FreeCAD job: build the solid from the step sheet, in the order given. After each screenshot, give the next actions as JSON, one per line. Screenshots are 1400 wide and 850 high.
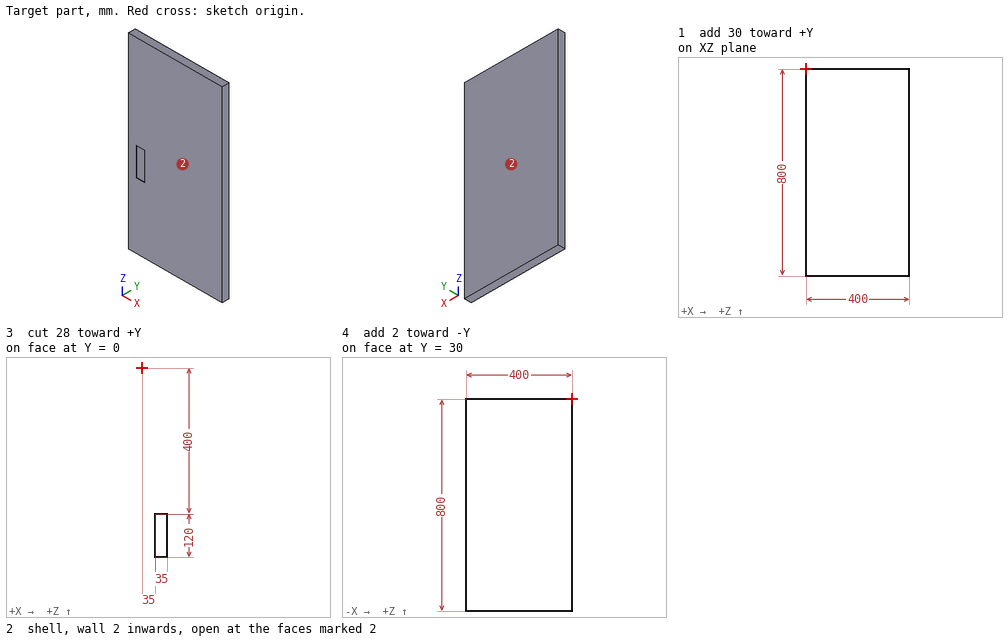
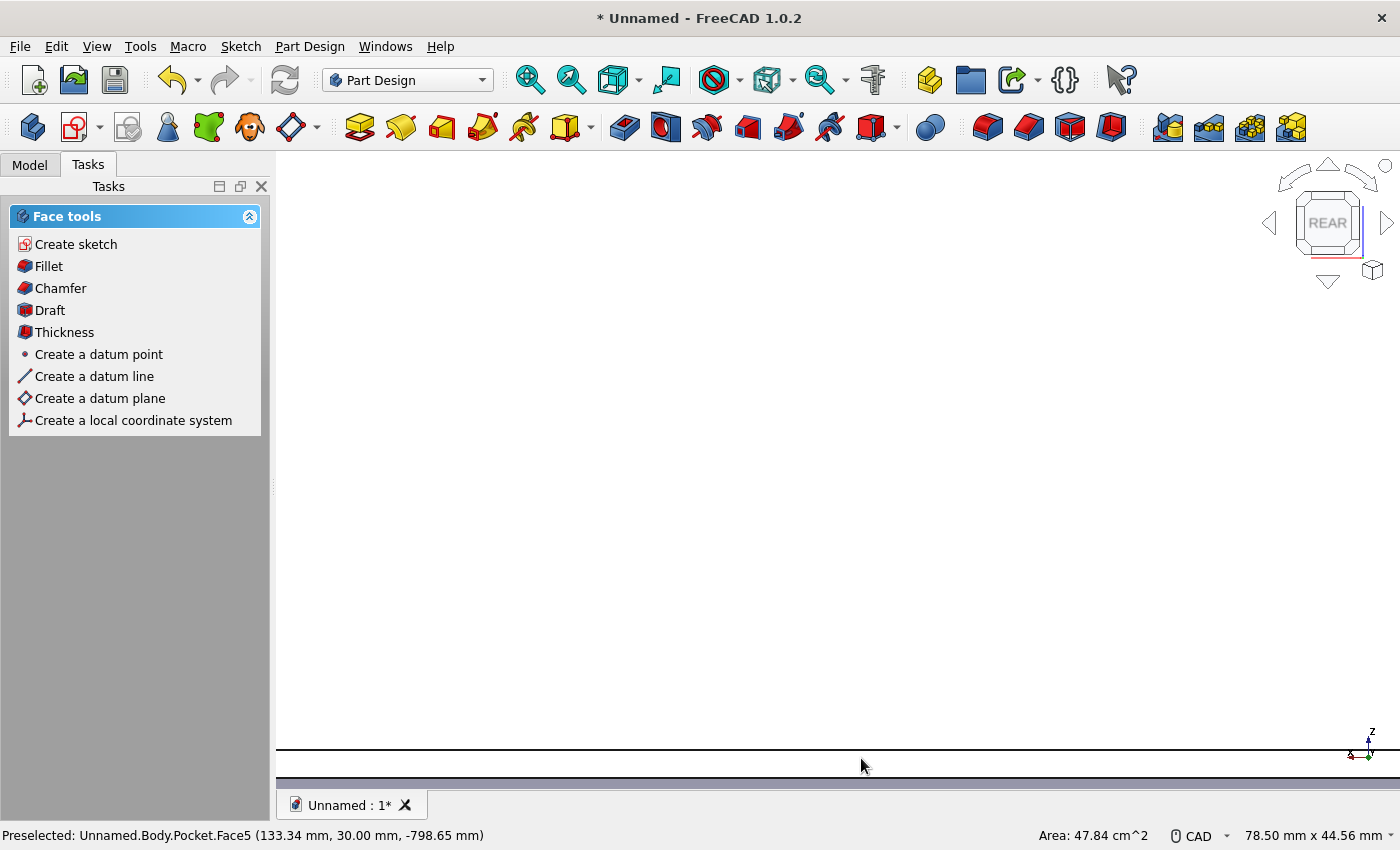
{"action": "left_click", "coordinate": [74, 128]}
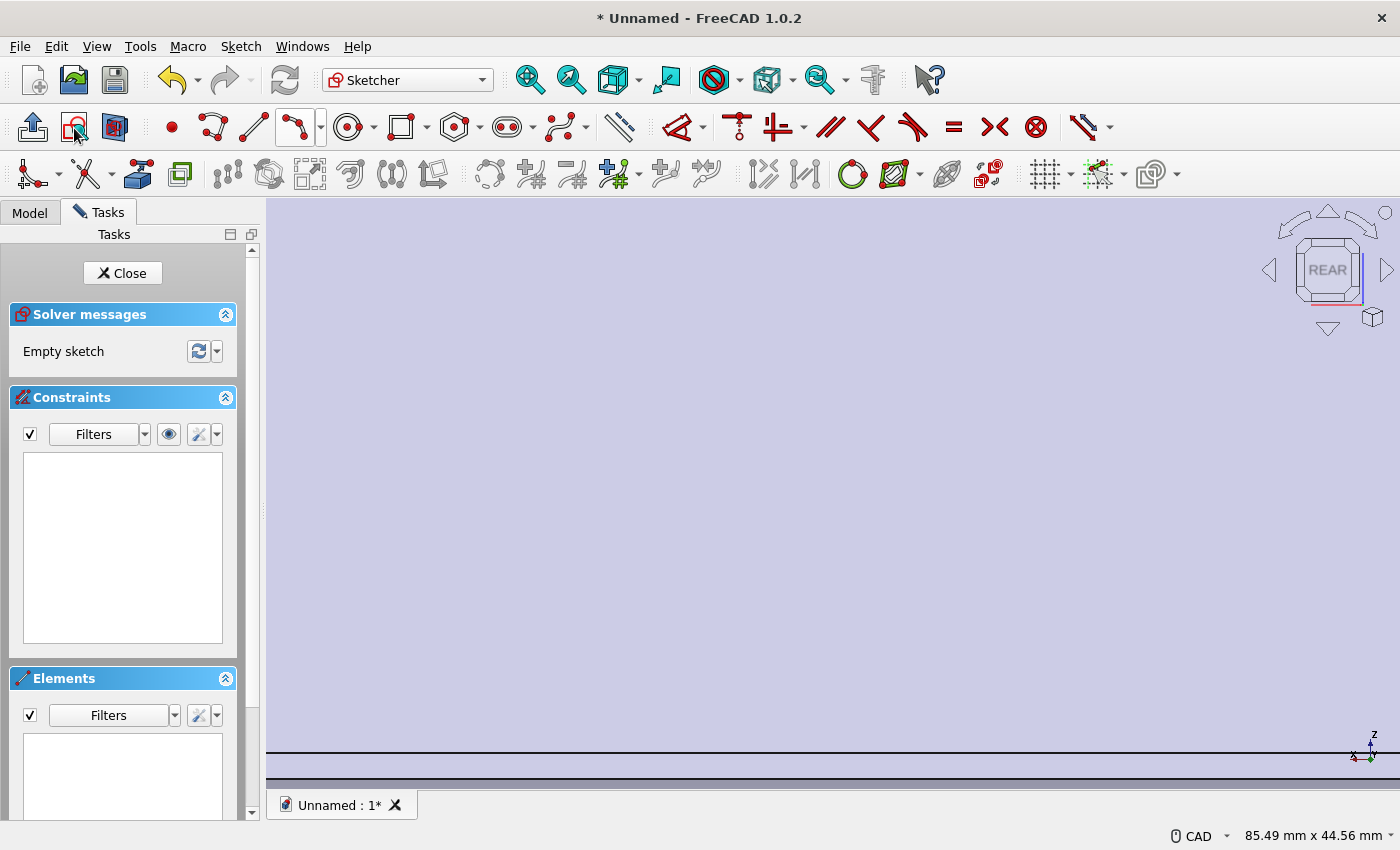
{"action": "scroll", "coordinate": [798, 707], "scroll_direction": "down", "scroll_amount": 16}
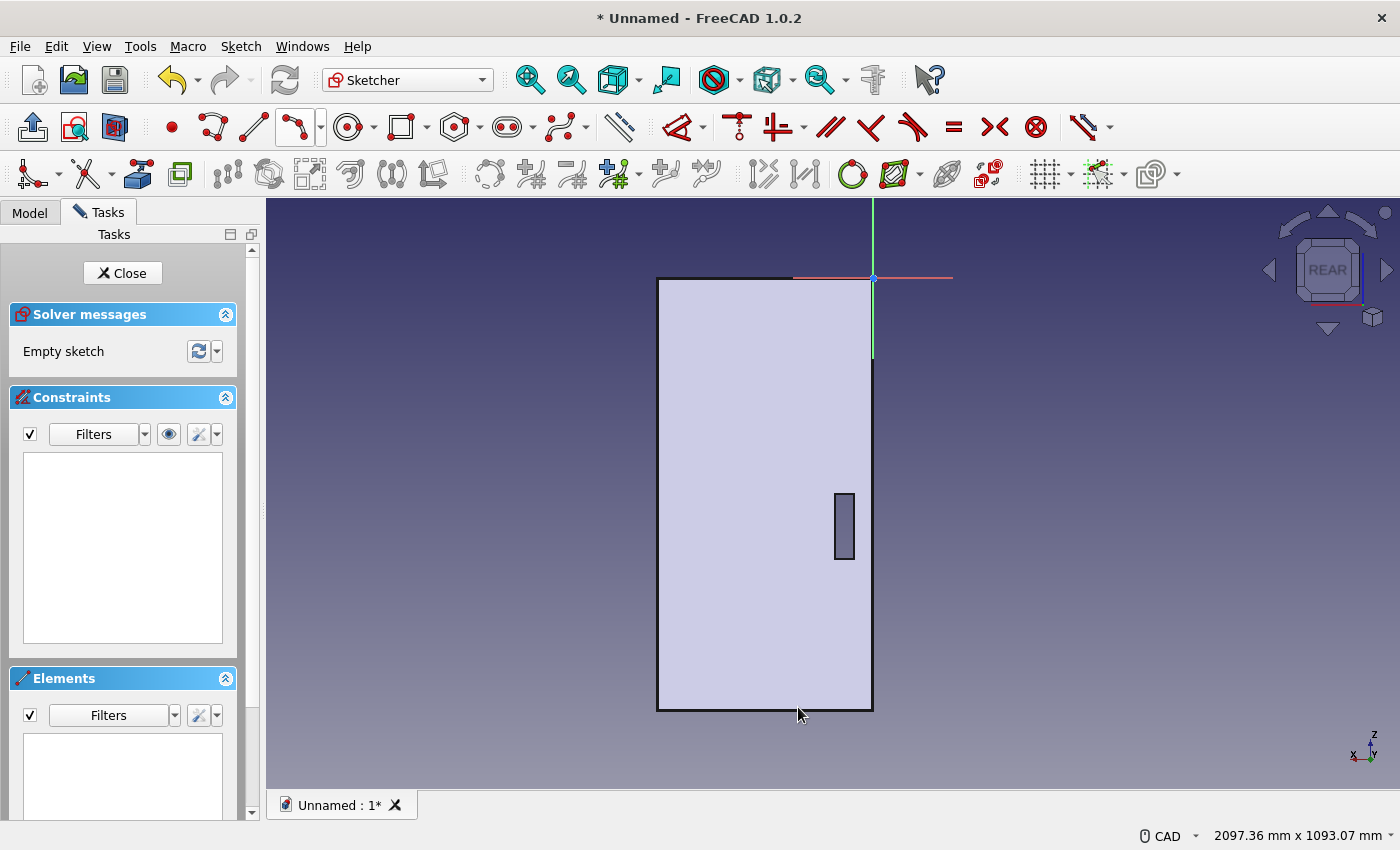
{"action": "key", "text": "g r"}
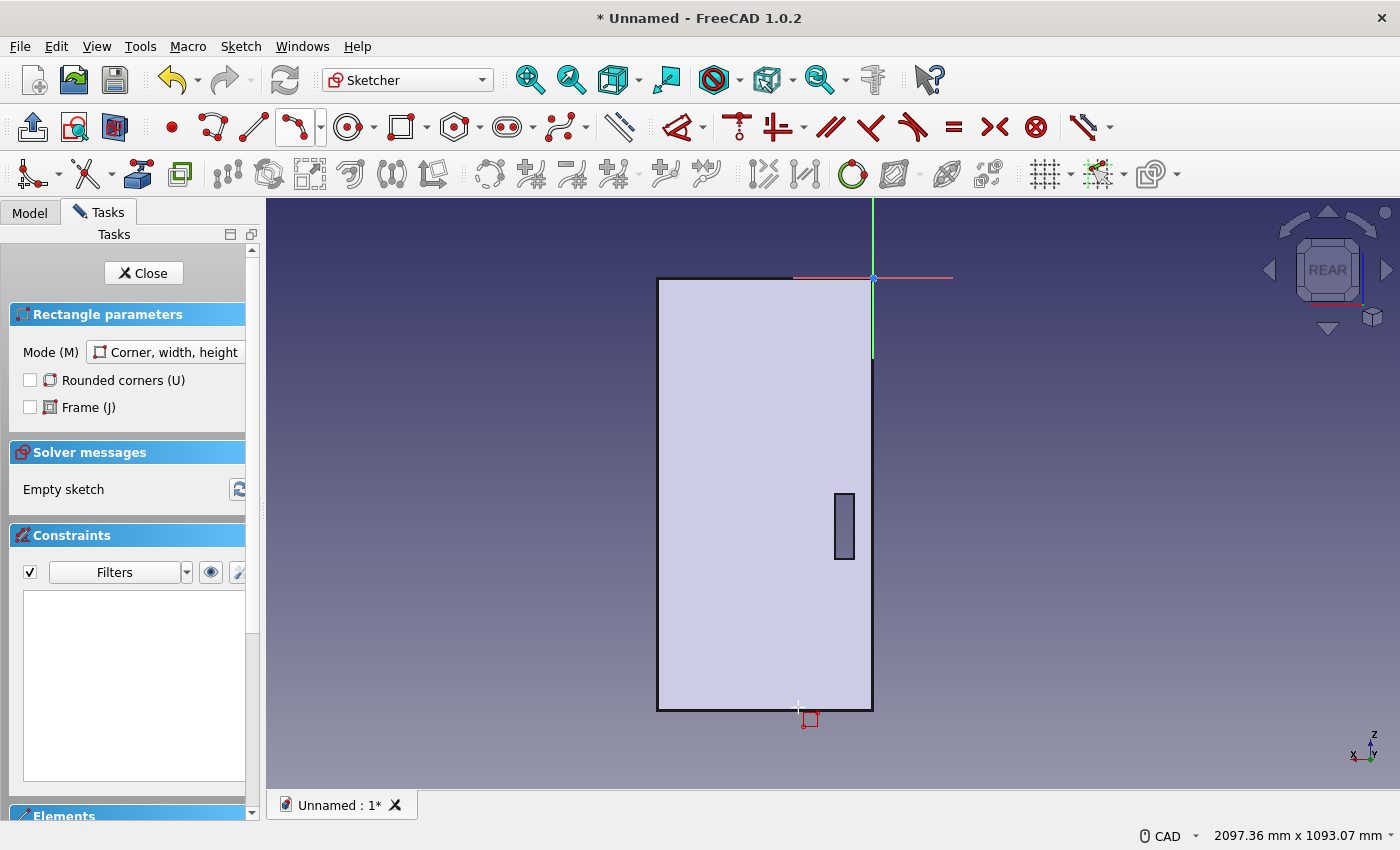
{"action": "left_click", "coordinate": [873, 278]}
{"action": "left_click", "coordinate": [657, 711]}
{"action": "key", "text": "Escape"}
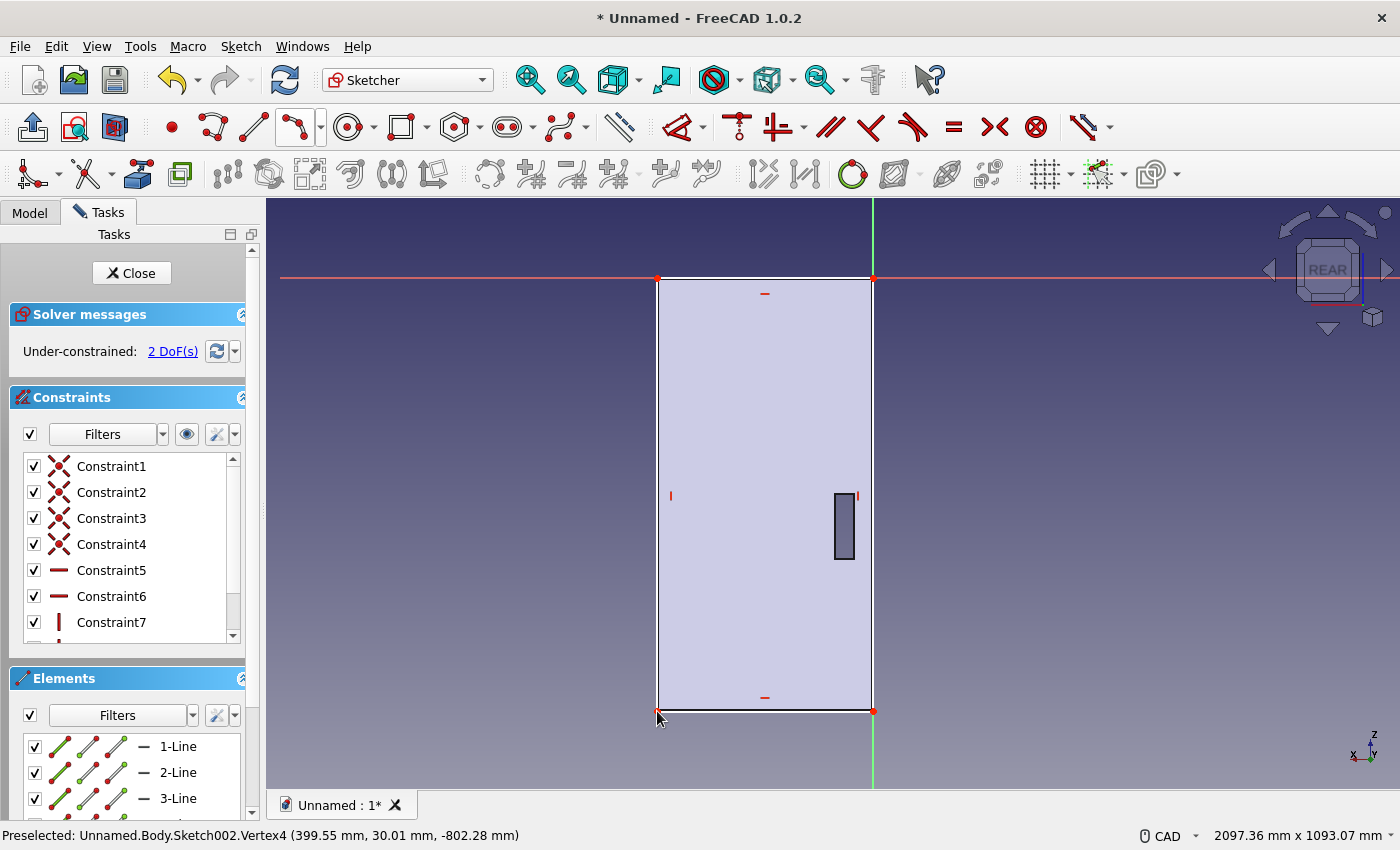
{"action": "left_click", "coordinate": [676, 128]}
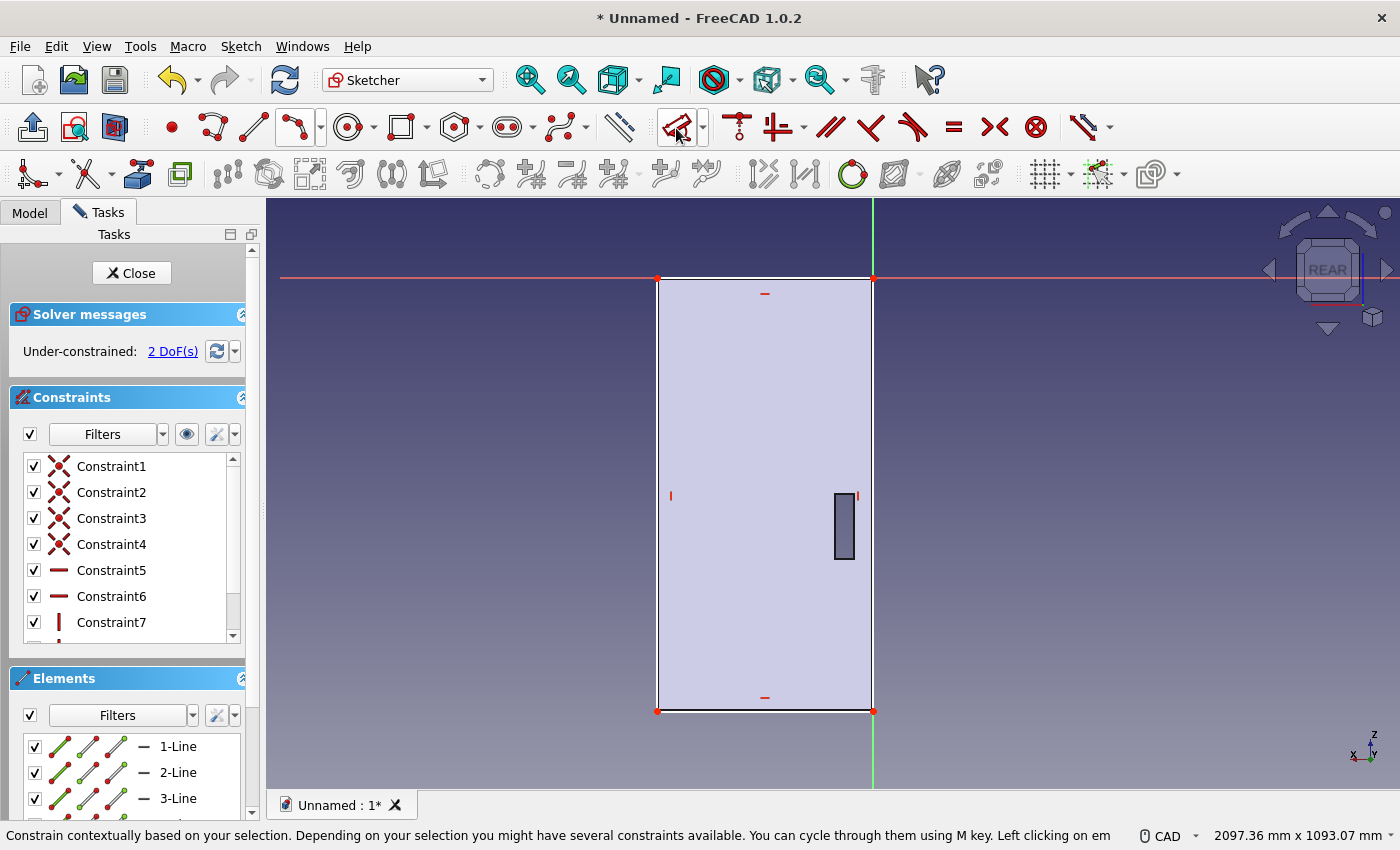
{"action": "left_click", "coordinate": [808, 278]}
{"action": "left_click", "coordinate": [765, 244]}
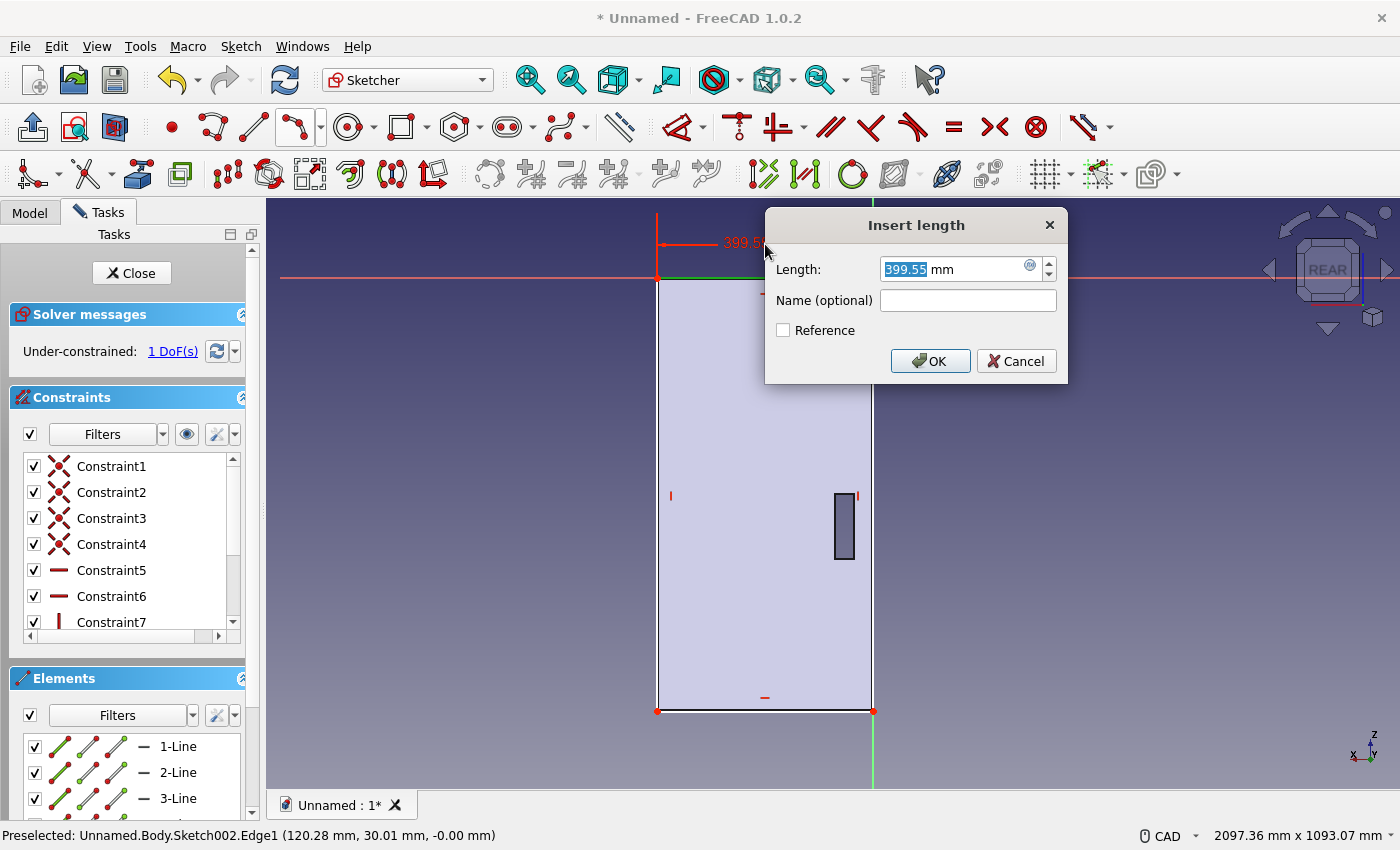
{"action": "type", "text": "400"}
{"action": "key", "text": "Return"}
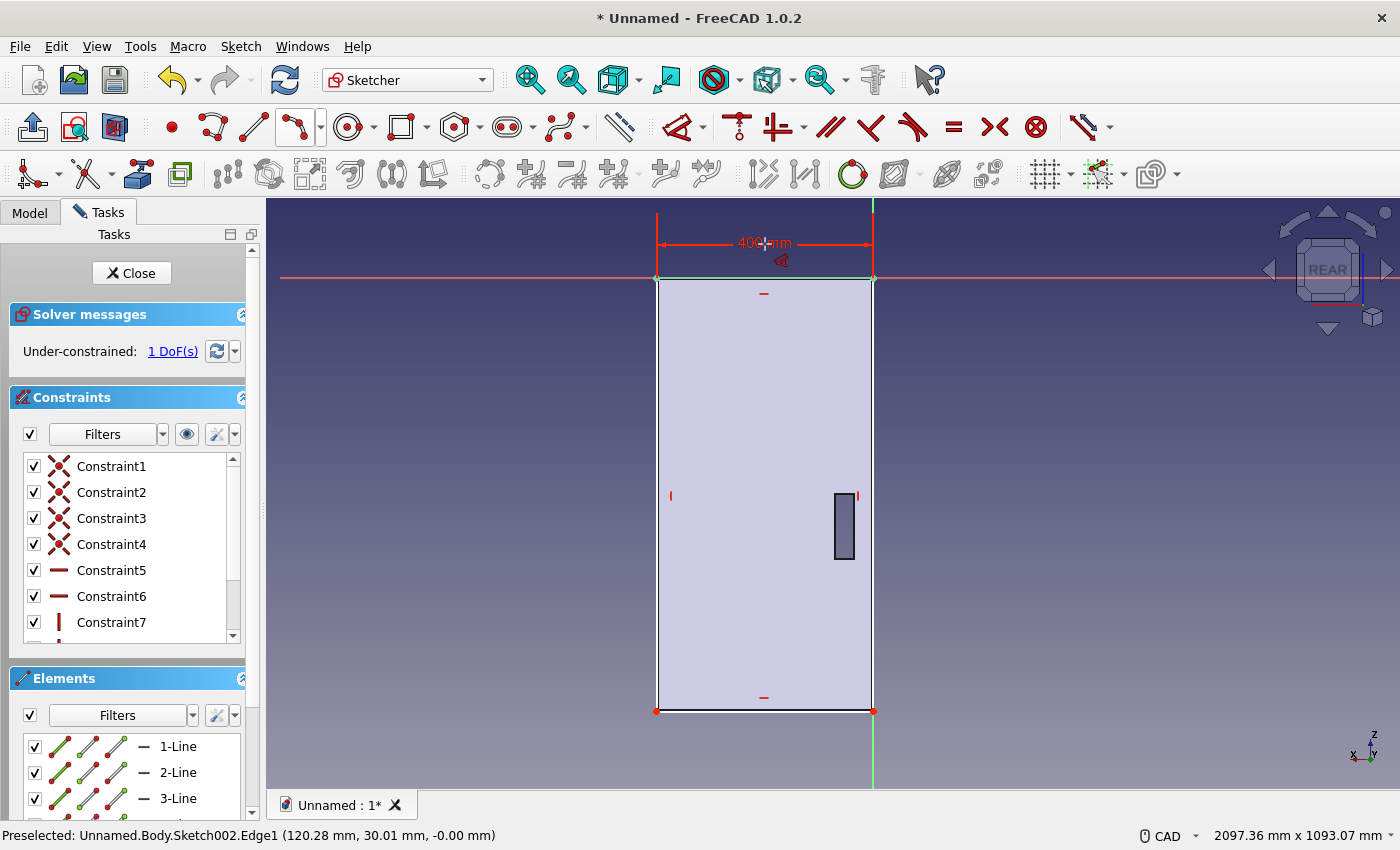
{"action": "left_click", "coordinate": [657, 408]}
{"action": "left_click", "coordinate": [623, 495]}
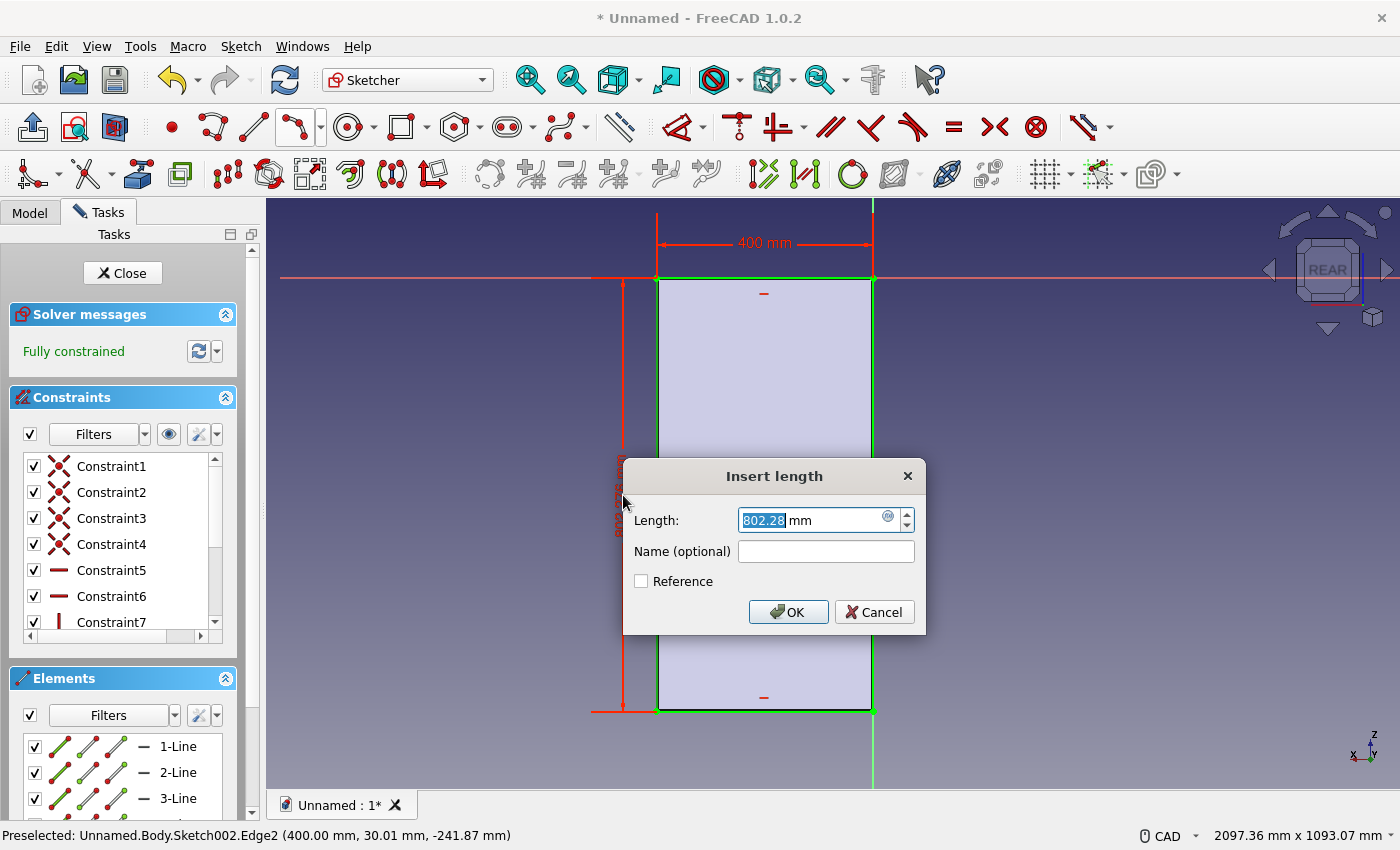
{"action": "type", "text": "800"}
{"action": "key", "text": "Return"}
{"action": "key", "text": "Escape"}